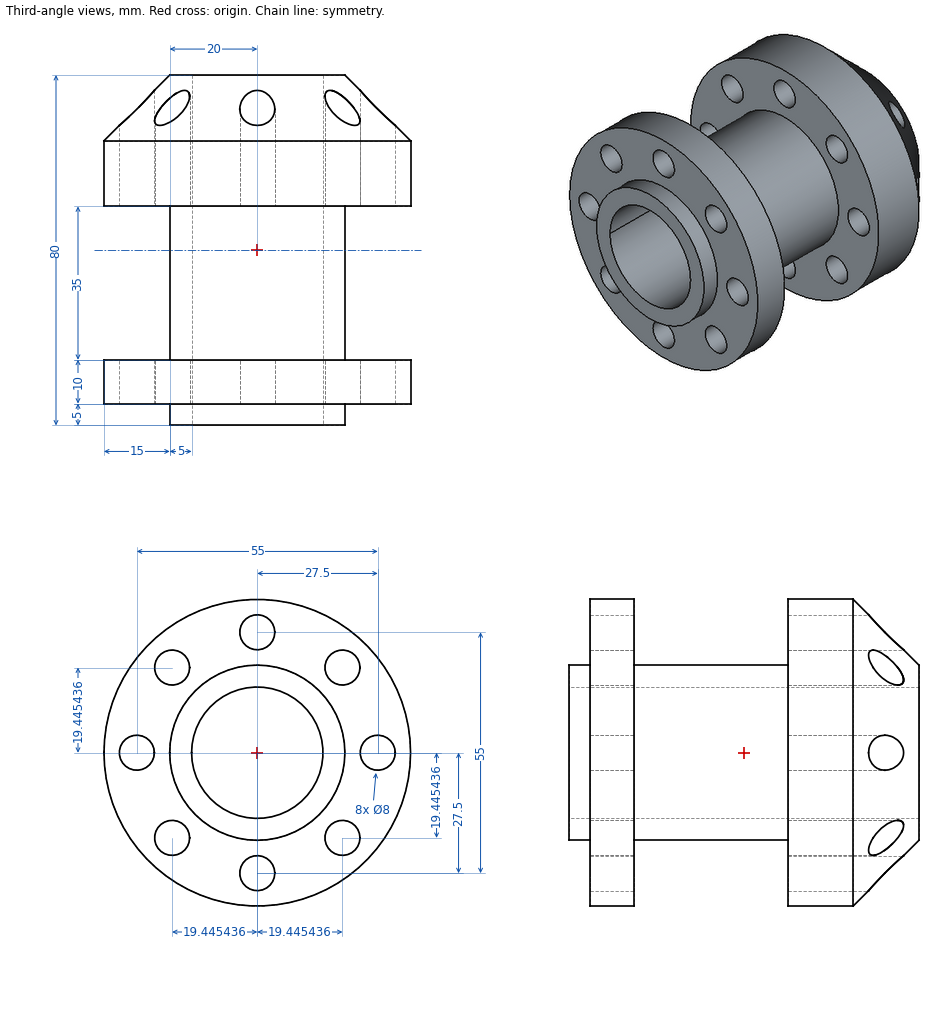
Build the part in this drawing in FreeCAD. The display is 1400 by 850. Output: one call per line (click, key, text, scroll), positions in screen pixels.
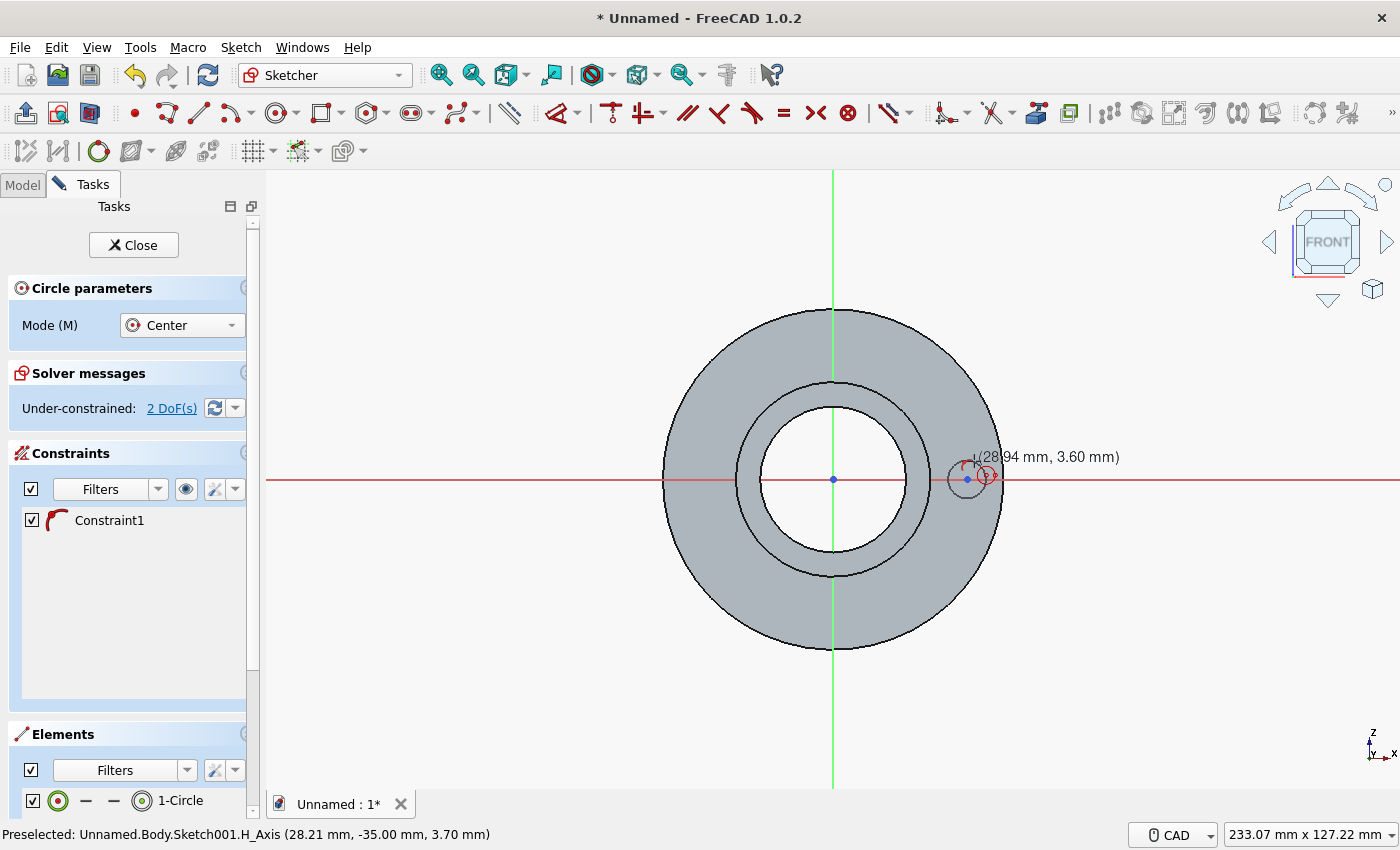
click(928, 574)
click(942, 560)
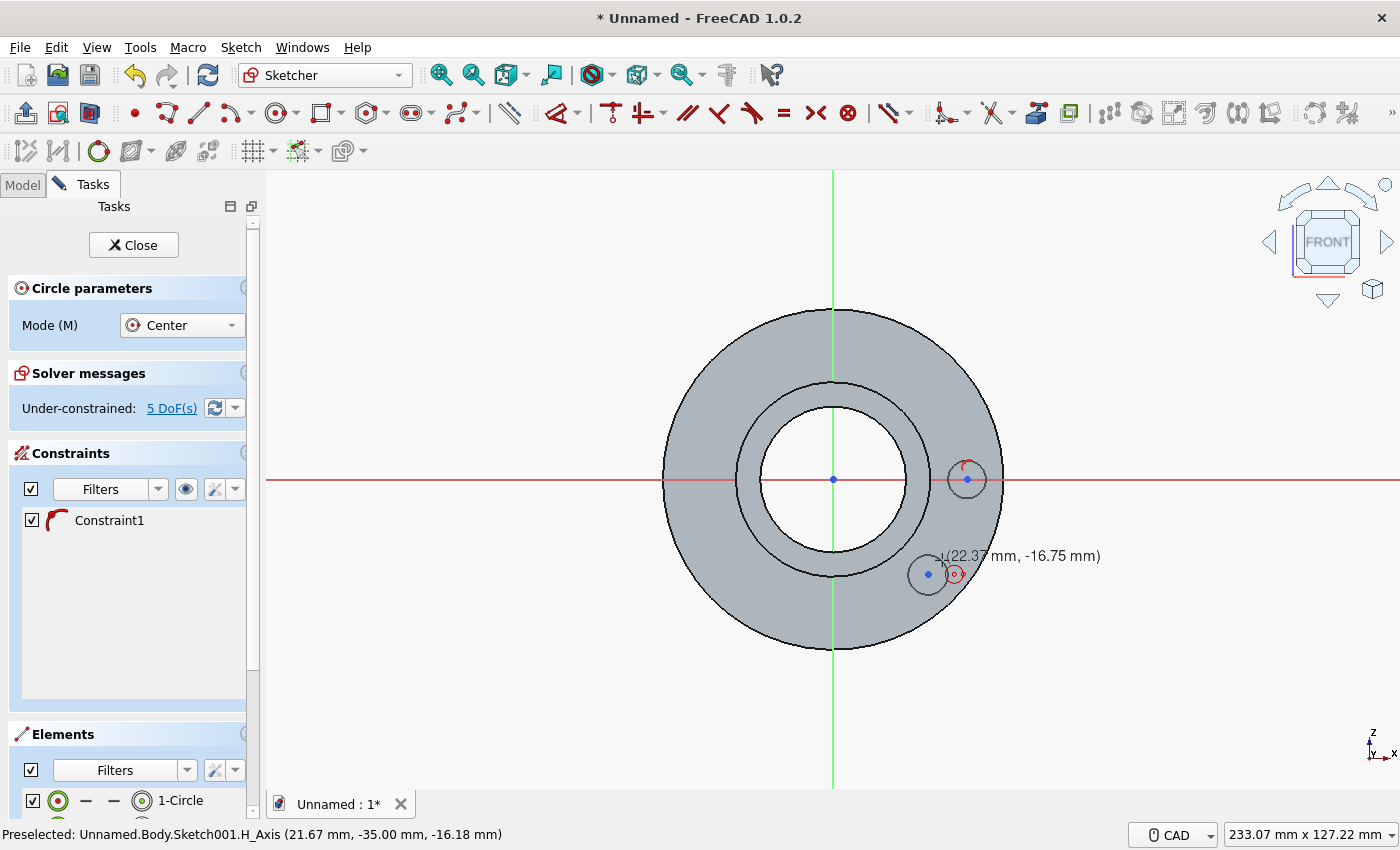
click(833, 613)
click(851, 607)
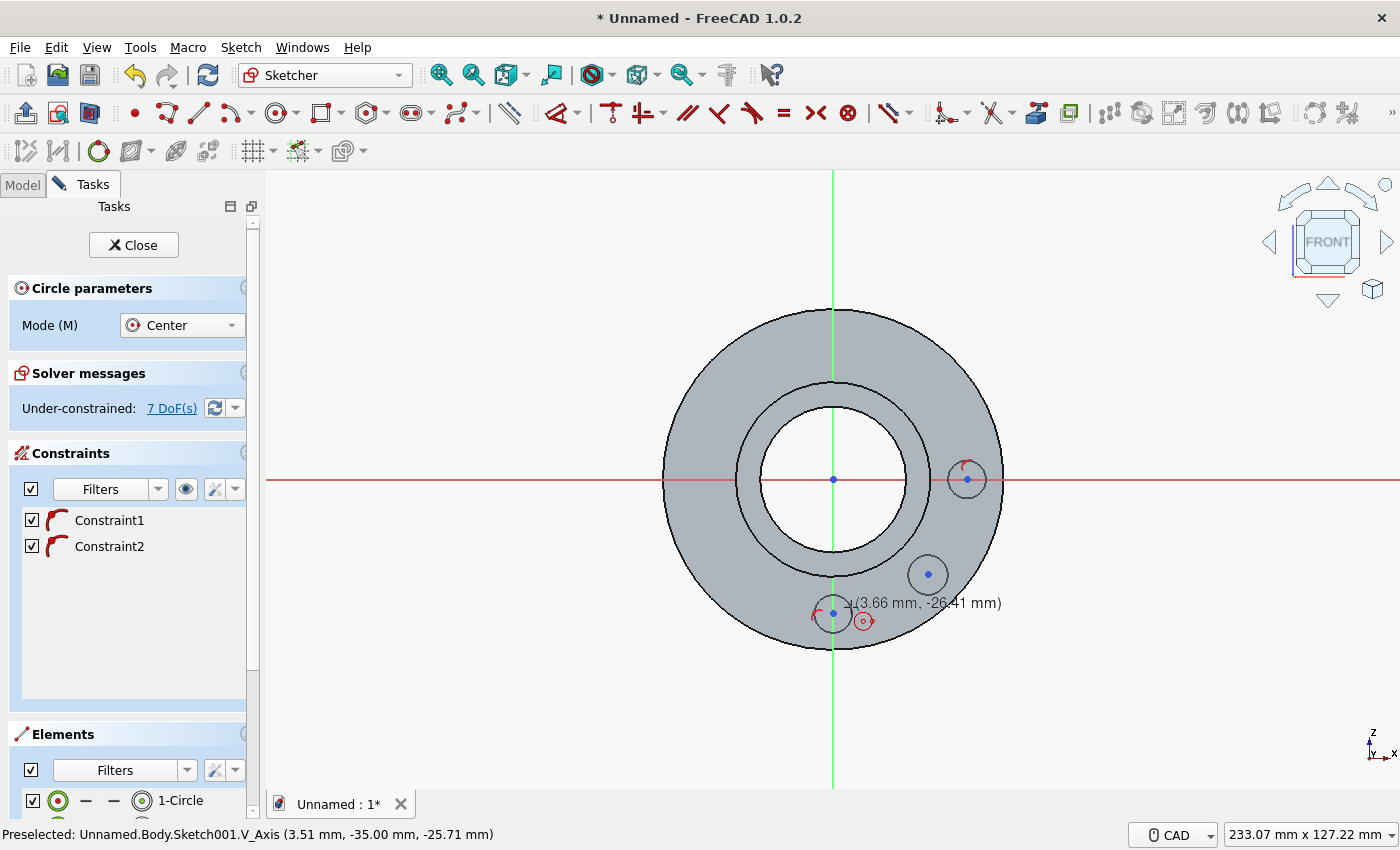
click(739, 574)
click(752, 560)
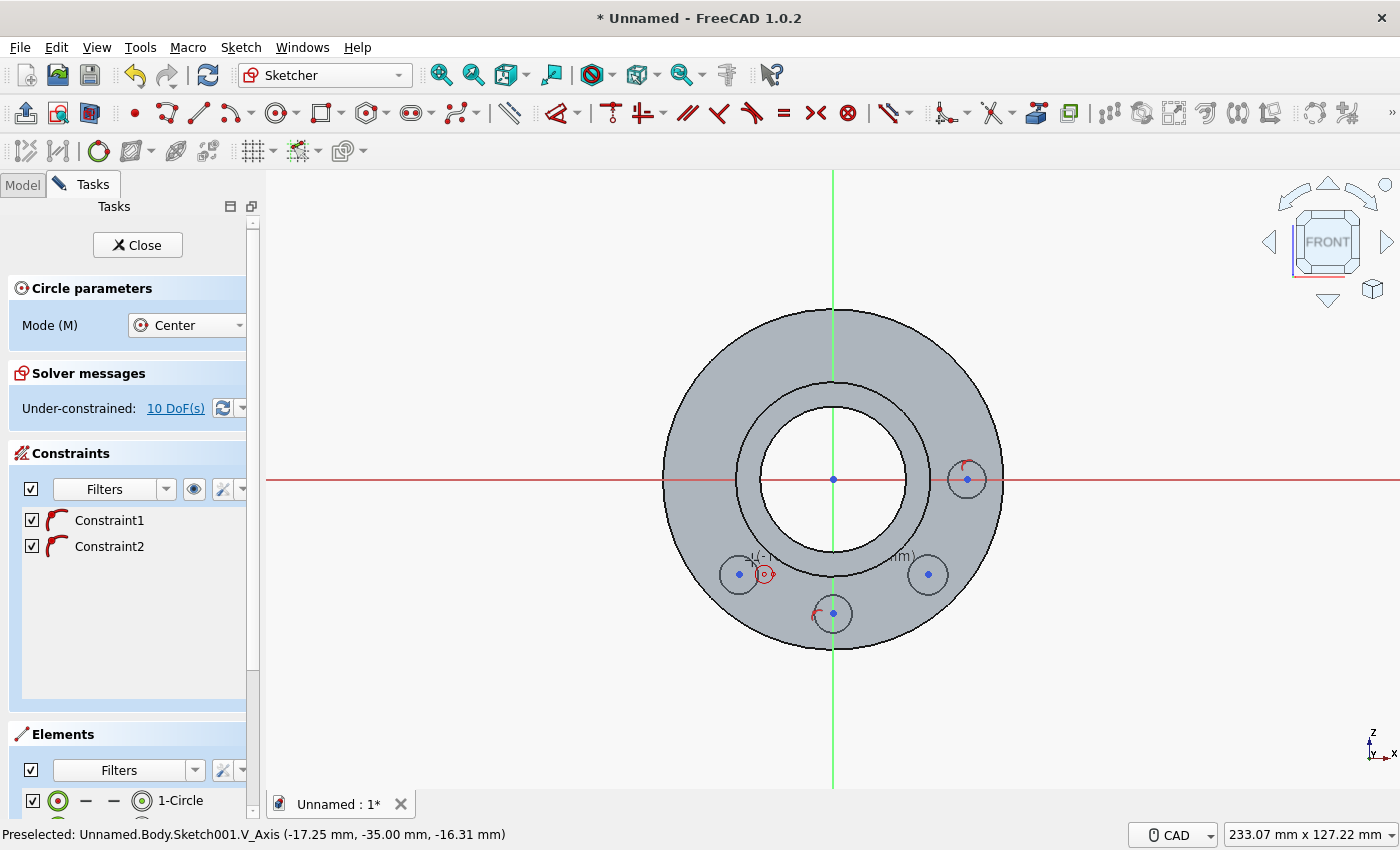
click(699, 480)
click(706, 461)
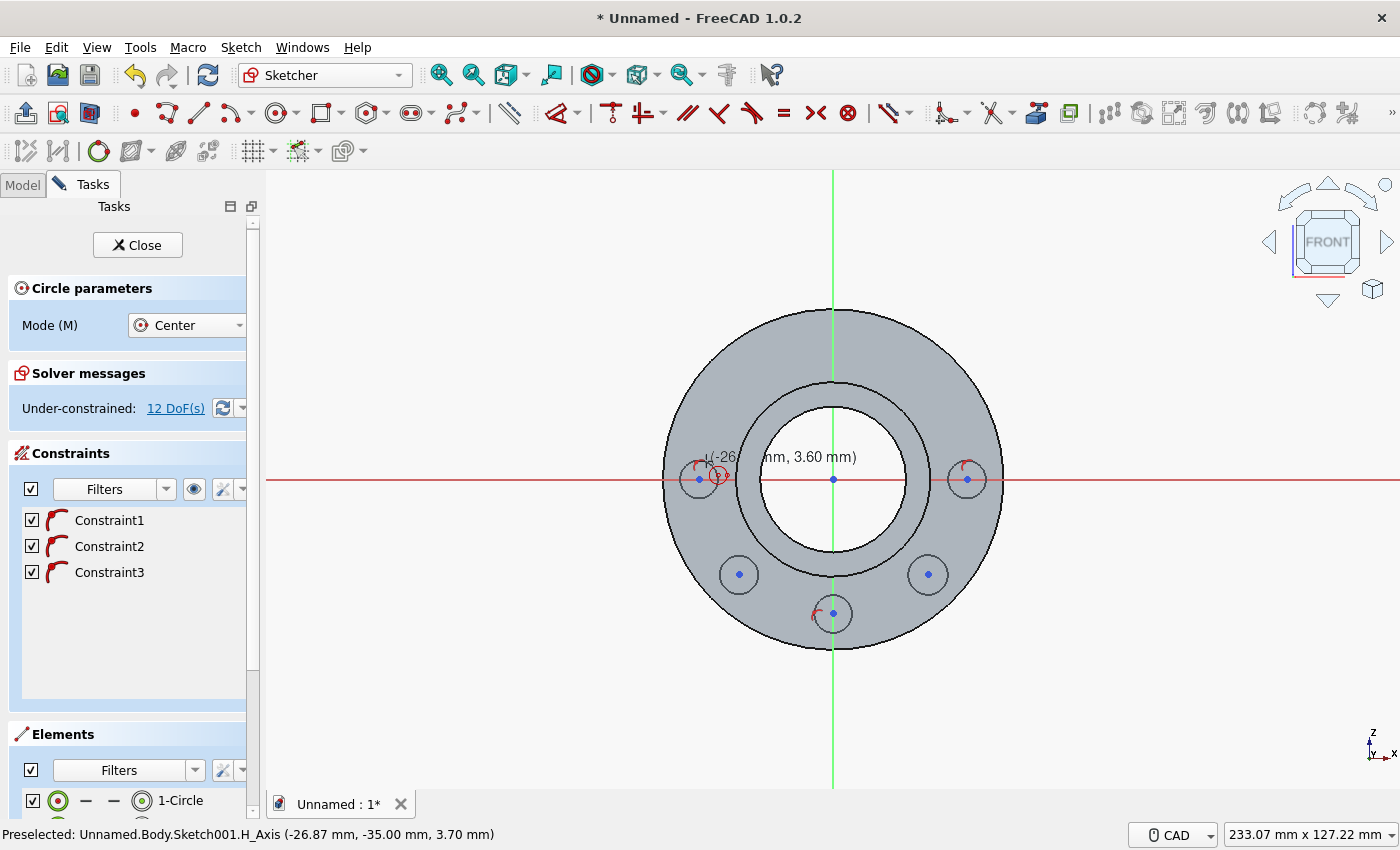
click(739, 385)
click(752, 371)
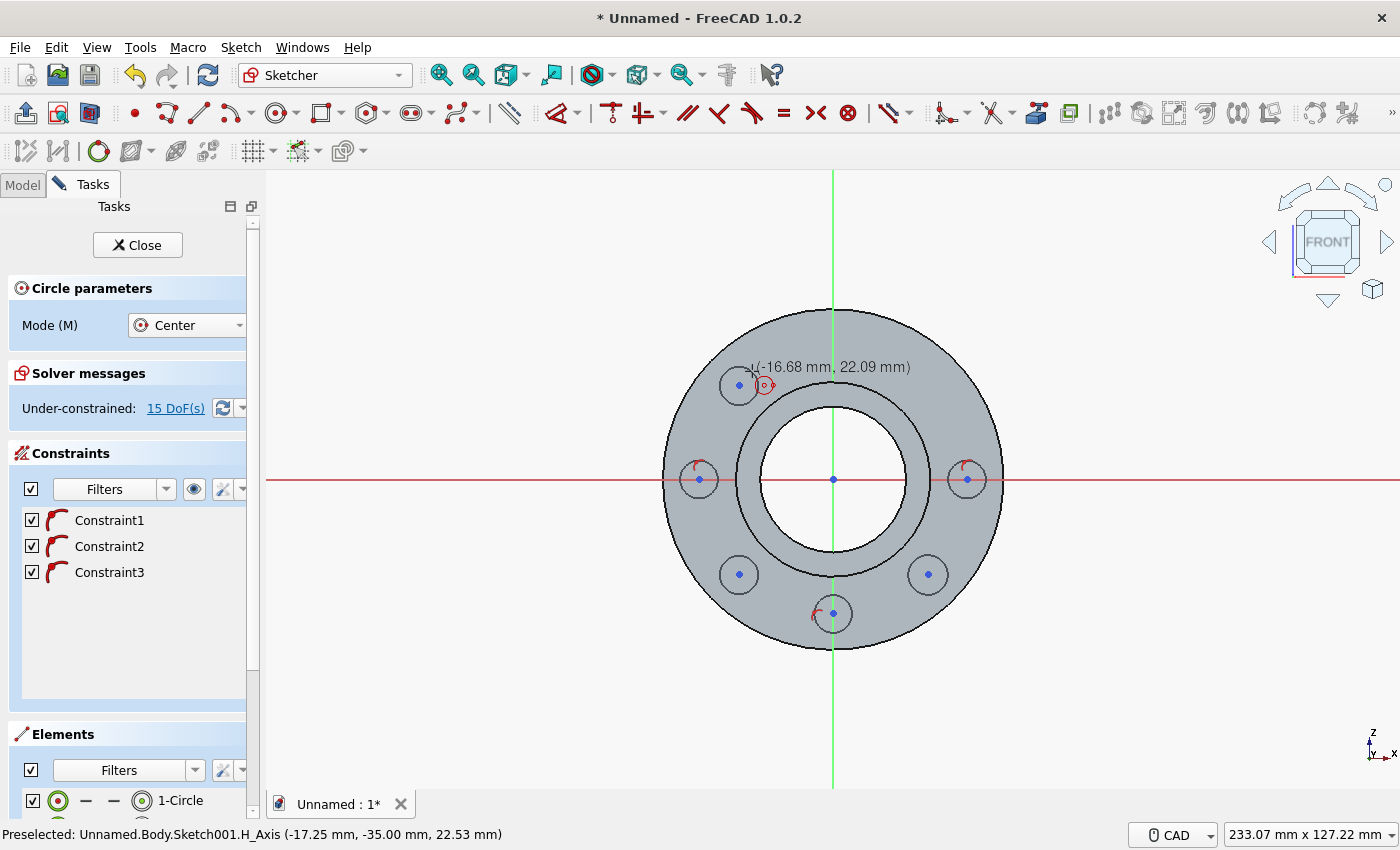
click(833, 346)
click(851, 339)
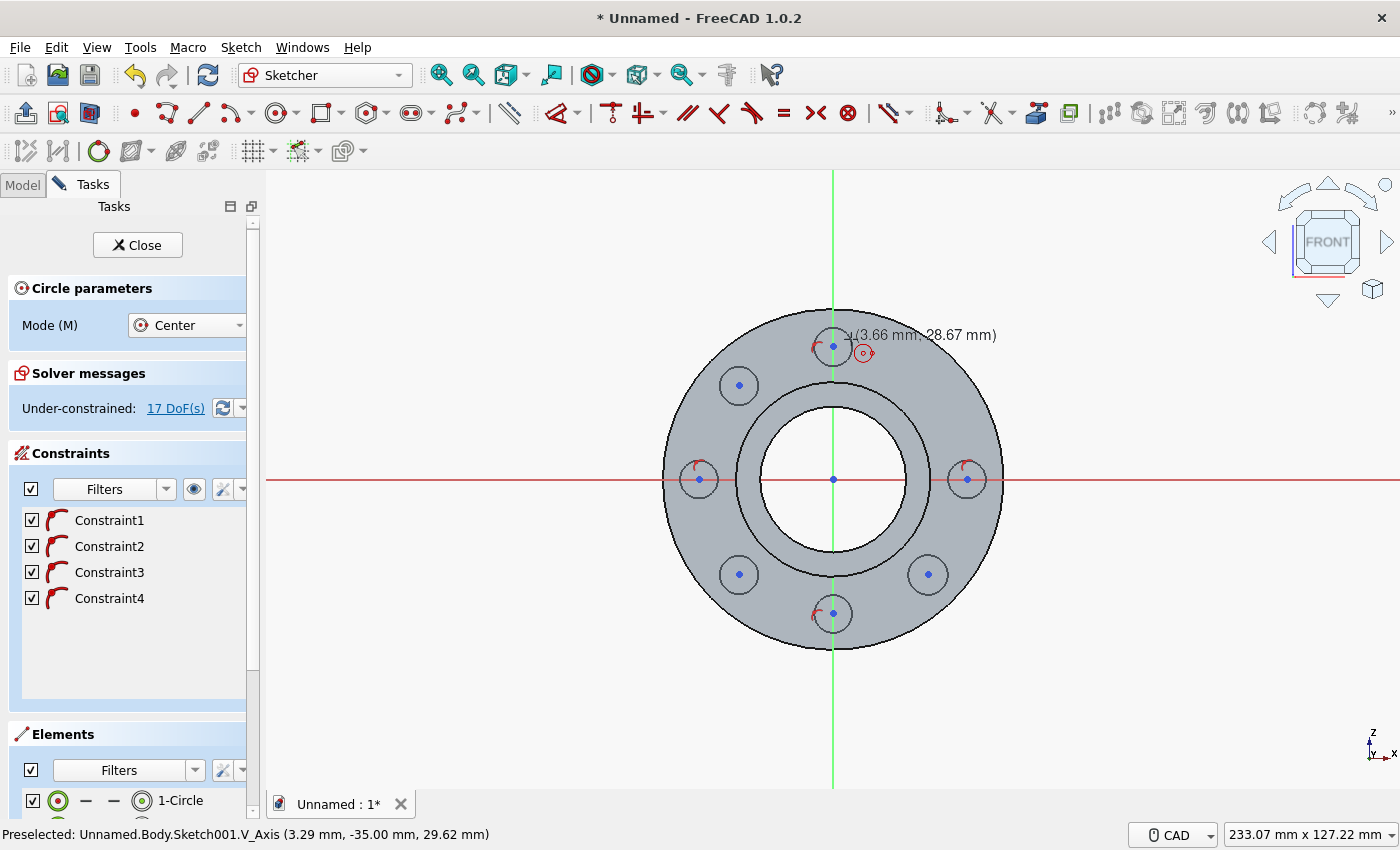
click(928, 385)
click(942, 371)
key(Escape)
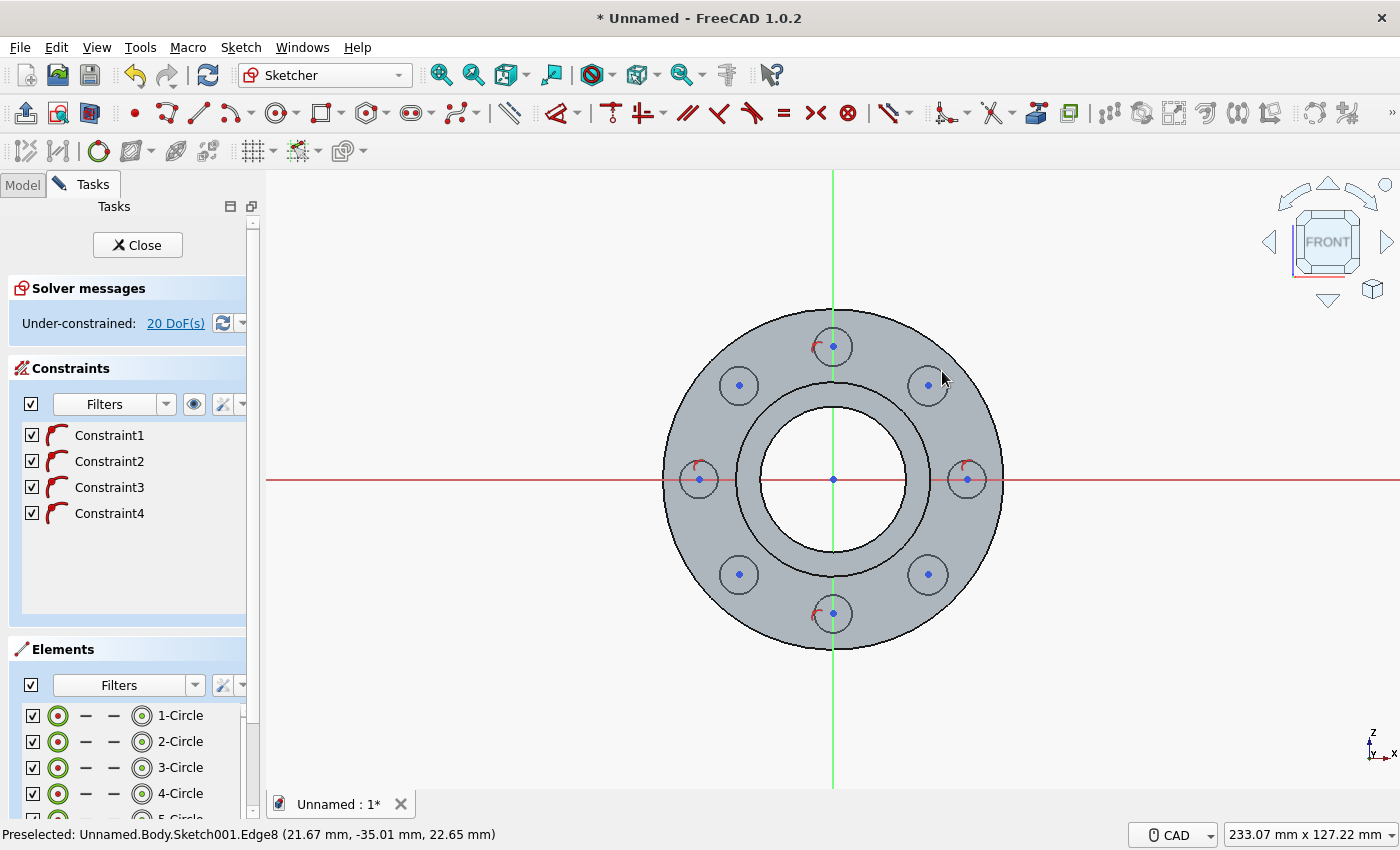
click(980, 466)